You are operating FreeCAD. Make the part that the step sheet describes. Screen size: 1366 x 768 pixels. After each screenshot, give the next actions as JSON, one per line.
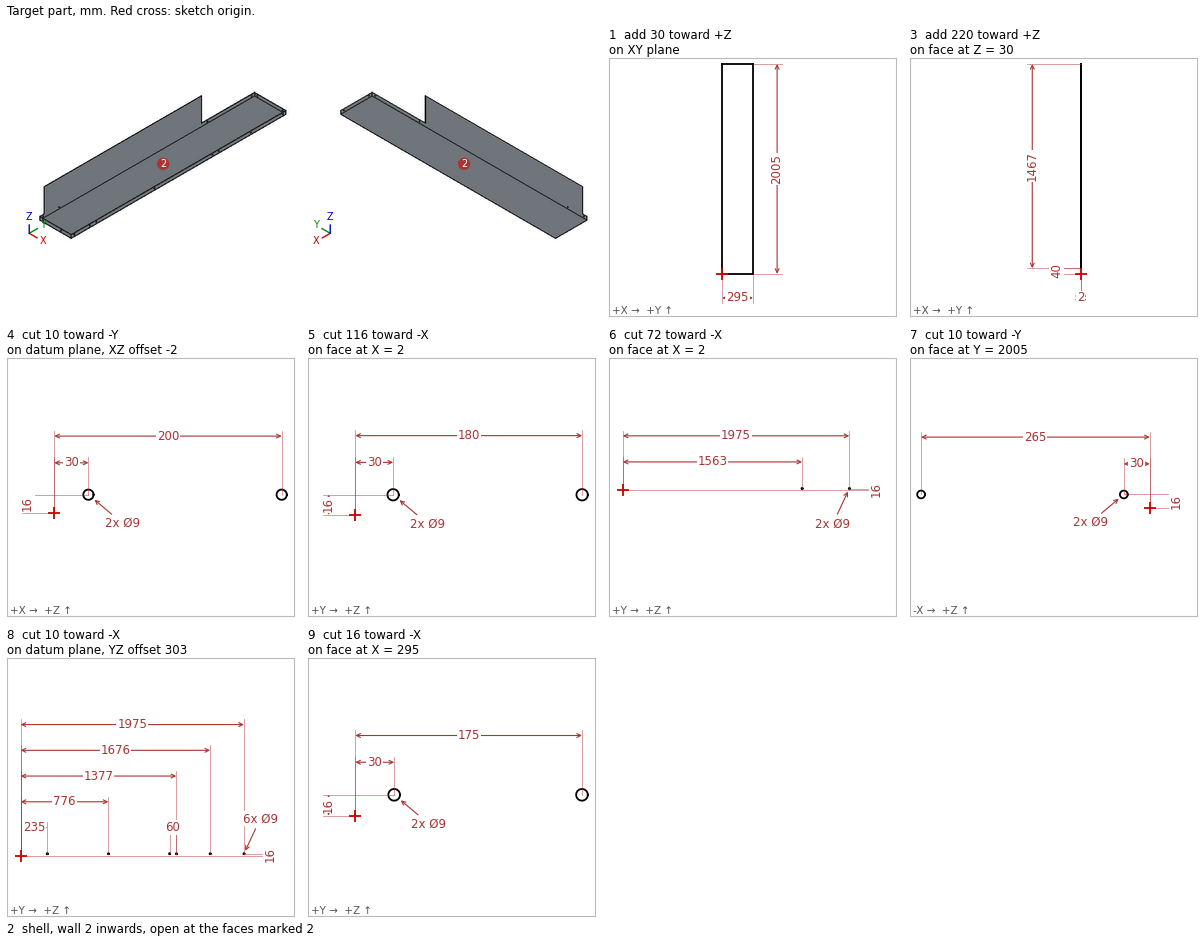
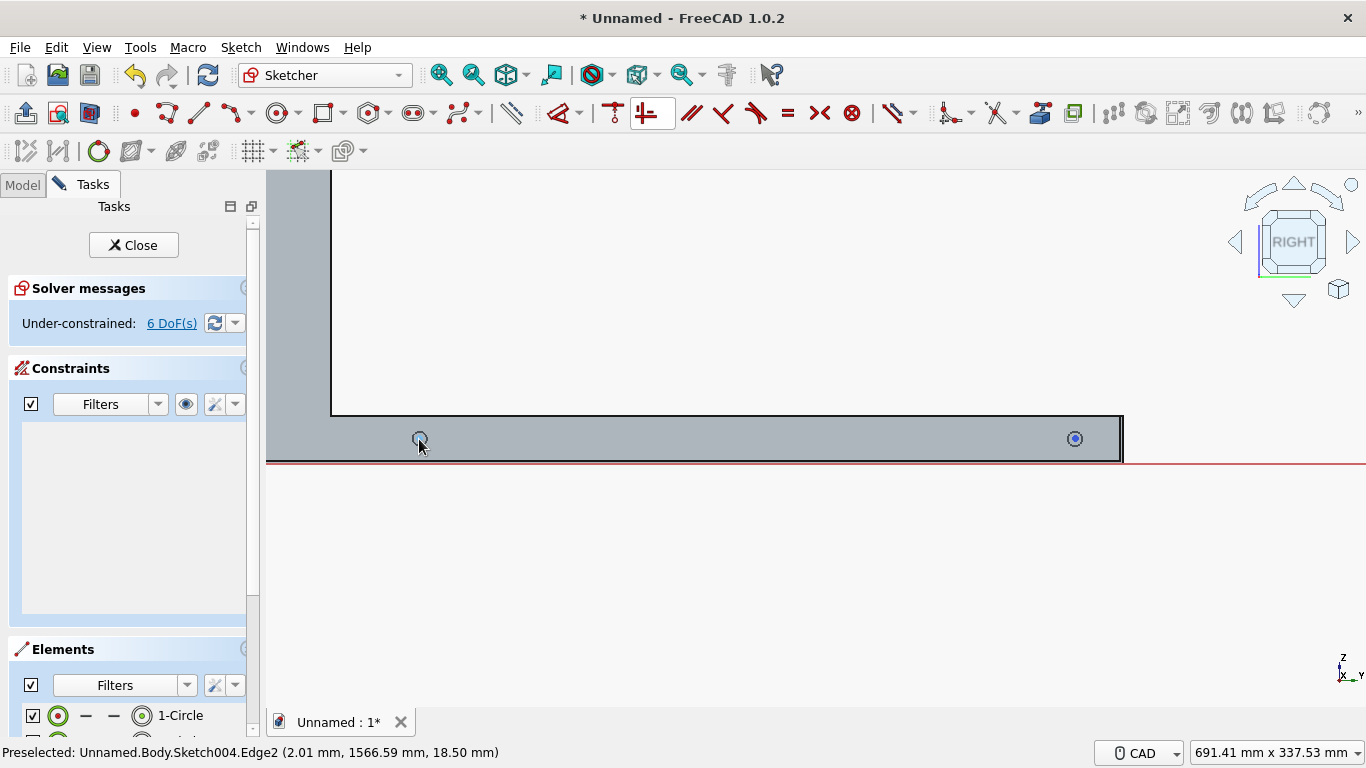
{"action": "scroll", "coordinate": [1080, 434], "scroll_direction": "up", "scroll_amount": 4}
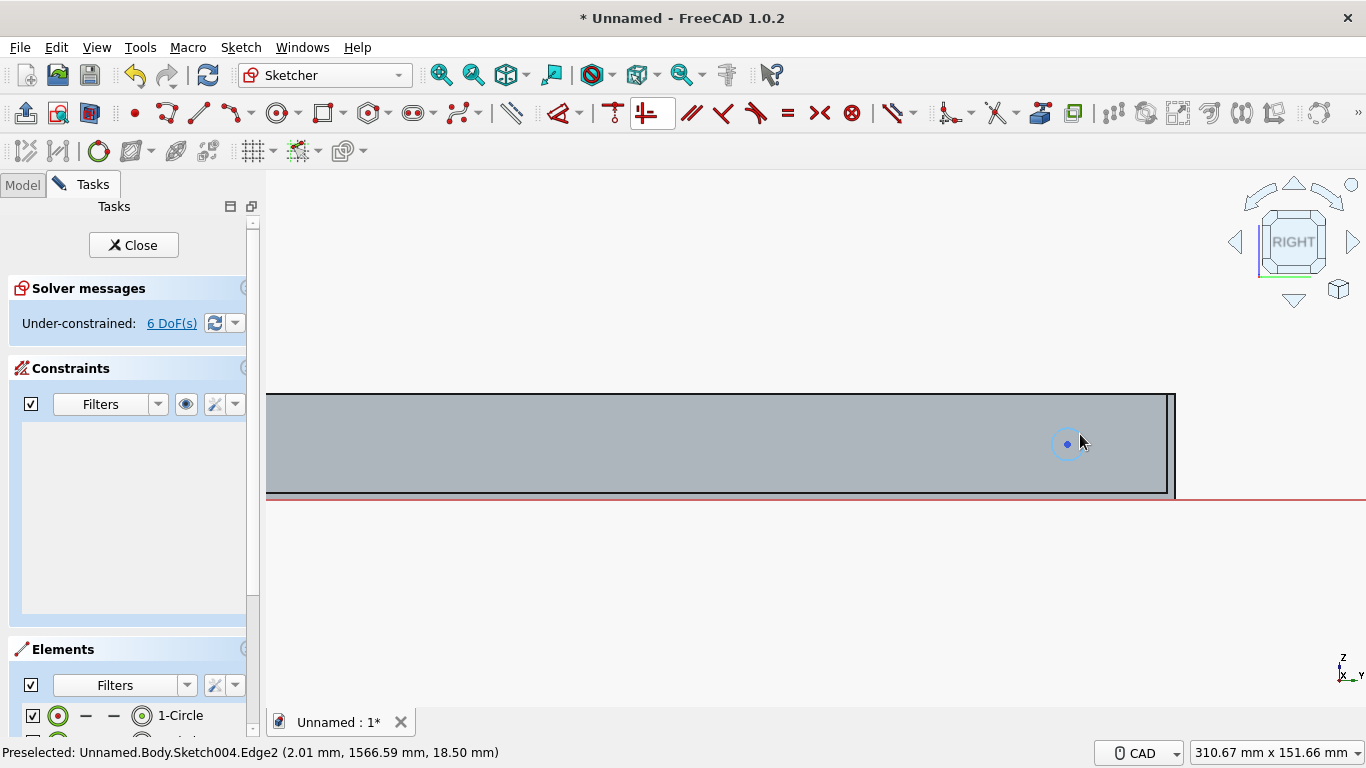
{"action": "left_click", "coordinate": [1079, 433]}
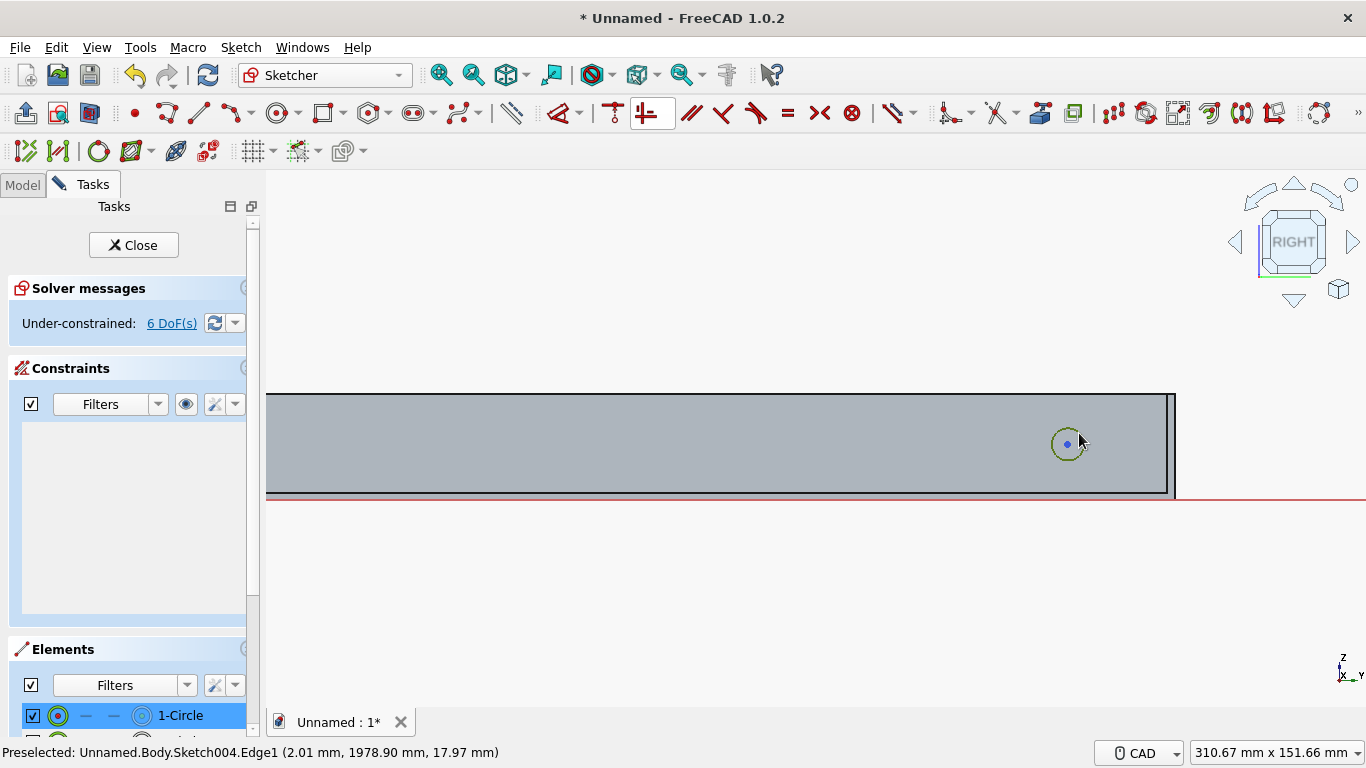
{"action": "scroll", "coordinate": [1081, 434], "scroll_direction": "down", "scroll_amount": 4}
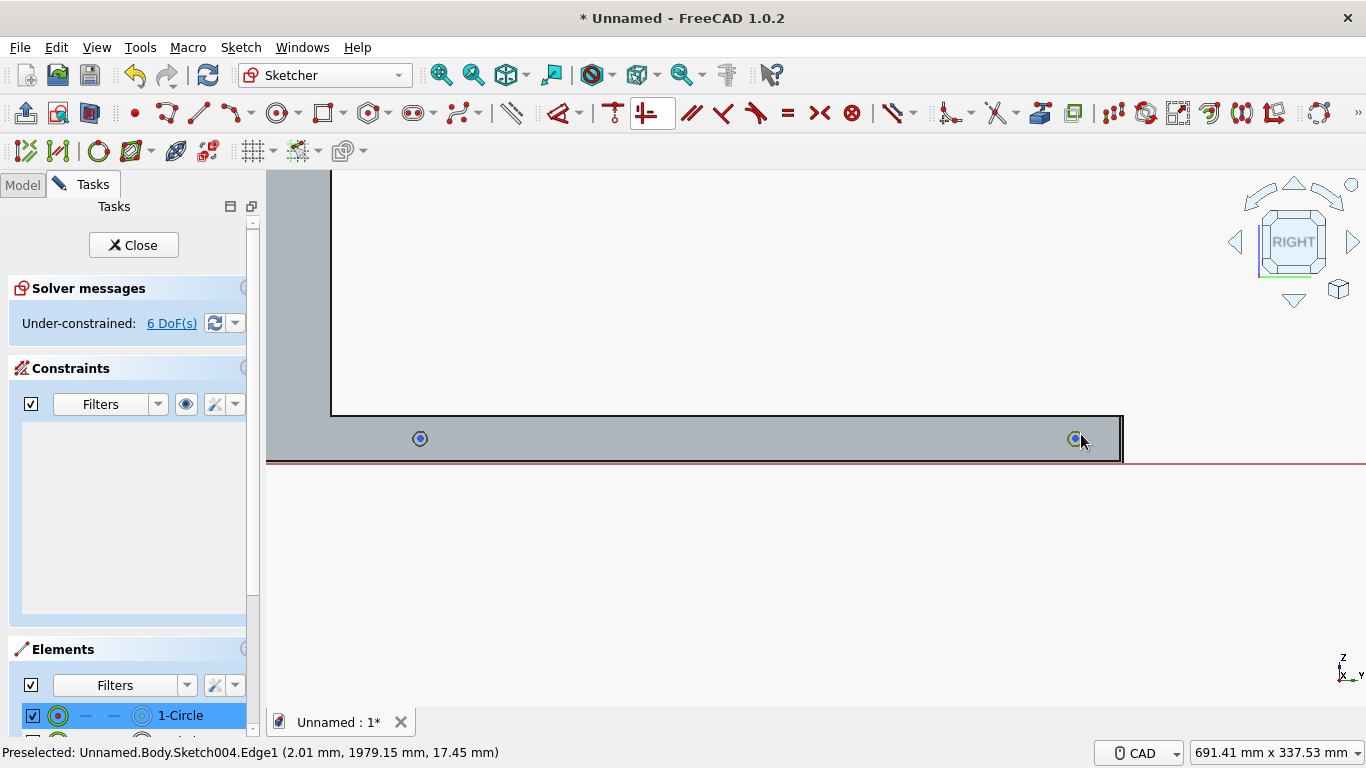
{"action": "scroll", "coordinate": [425, 434], "scroll_direction": "up", "scroll_amount": 4}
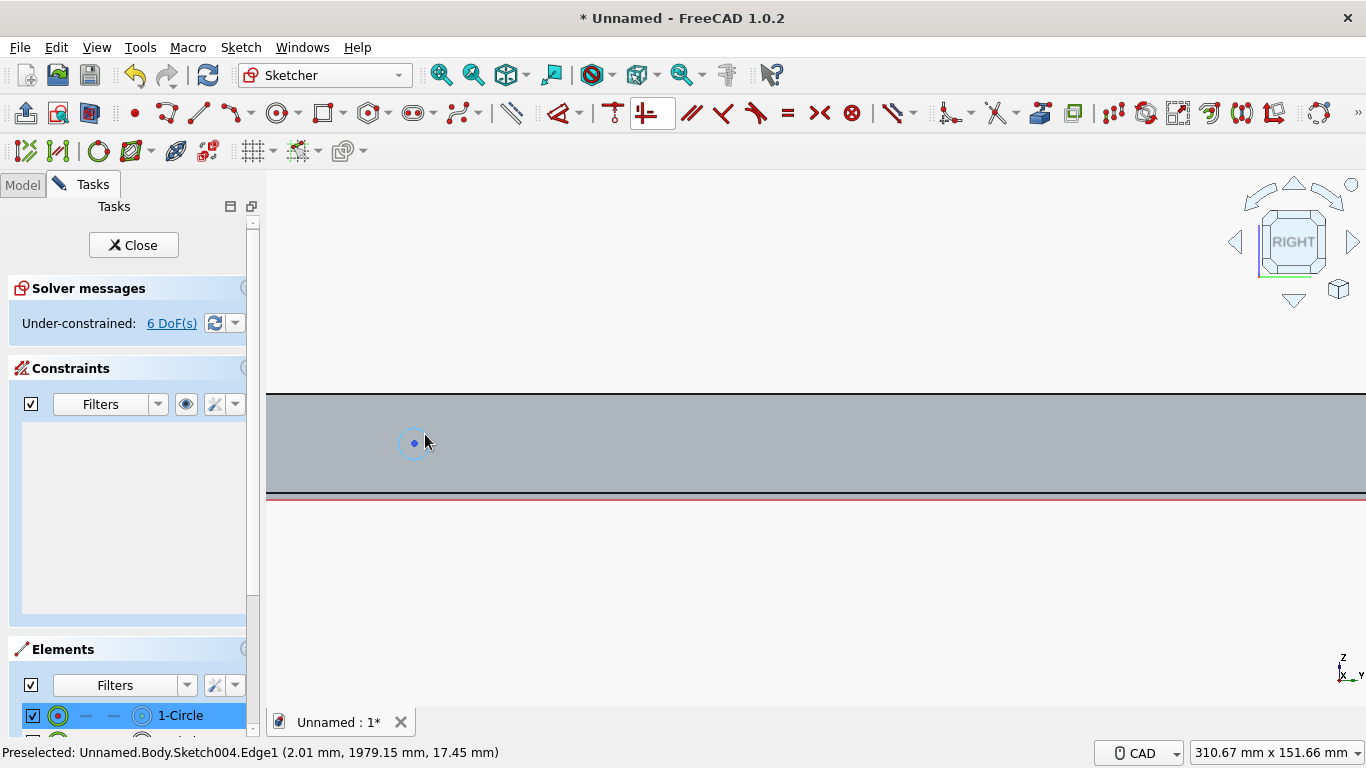
{"action": "left_click", "coordinate": [425, 433]}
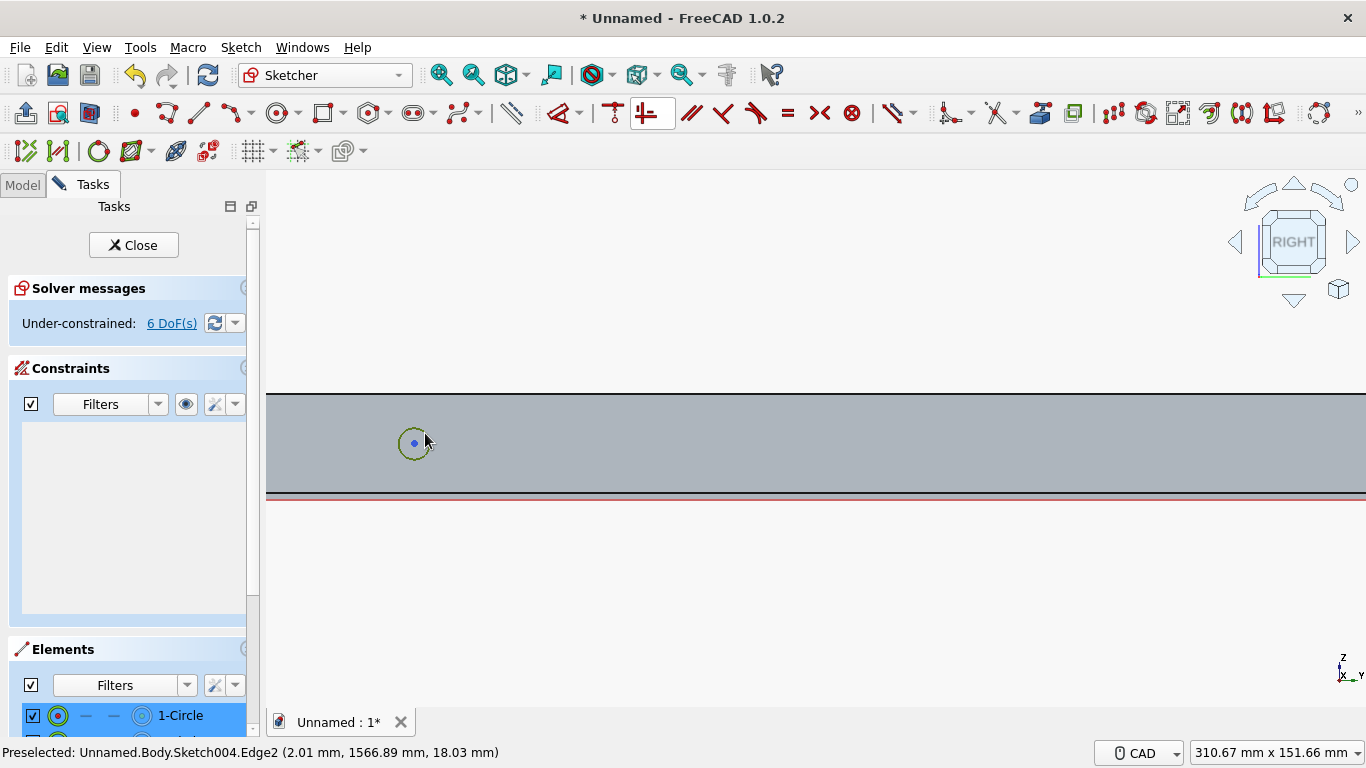
{"action": "left_click", "coordinate": [788, 114]}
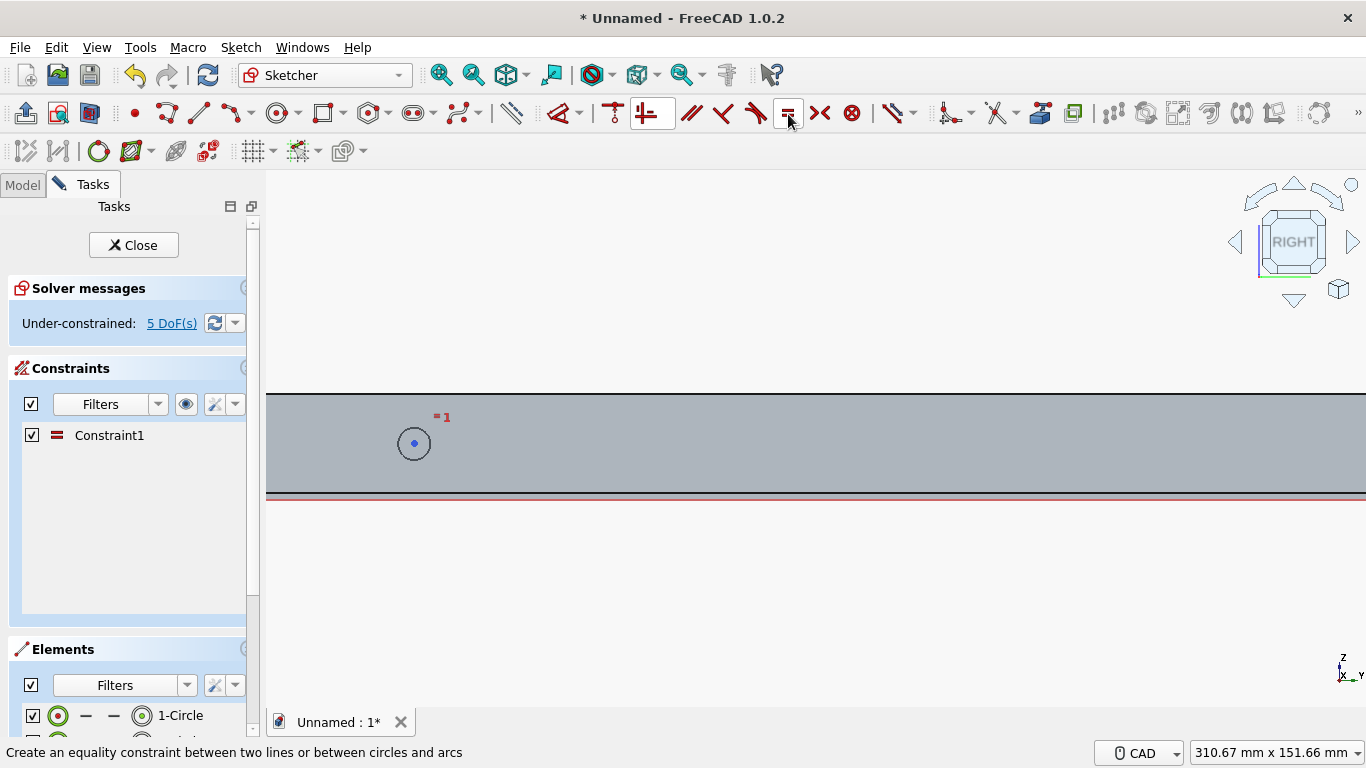
{"action": "scroll", "coordinate": [424, 434], "scroll_direction": "down", "scroll_amount": 4}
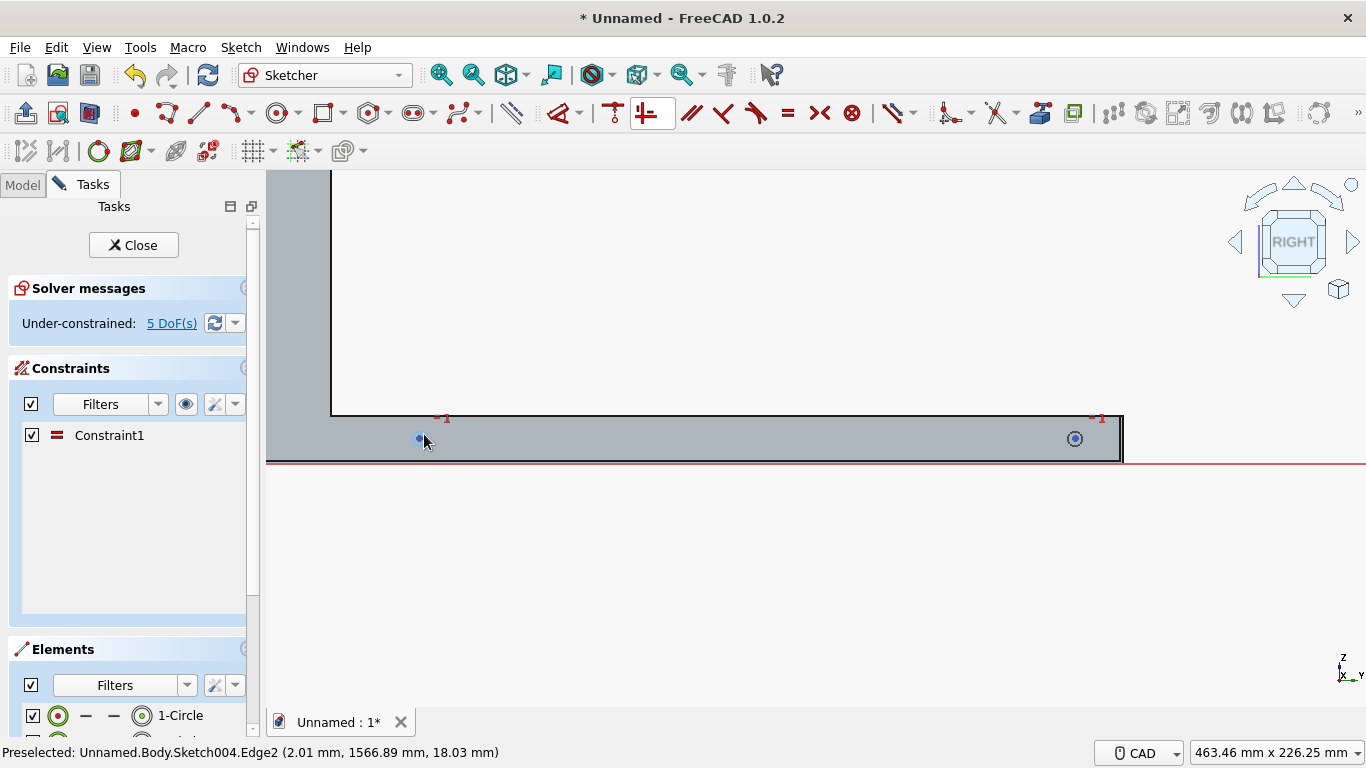
{"action": "left_click", "coordinate": [1075, 439]}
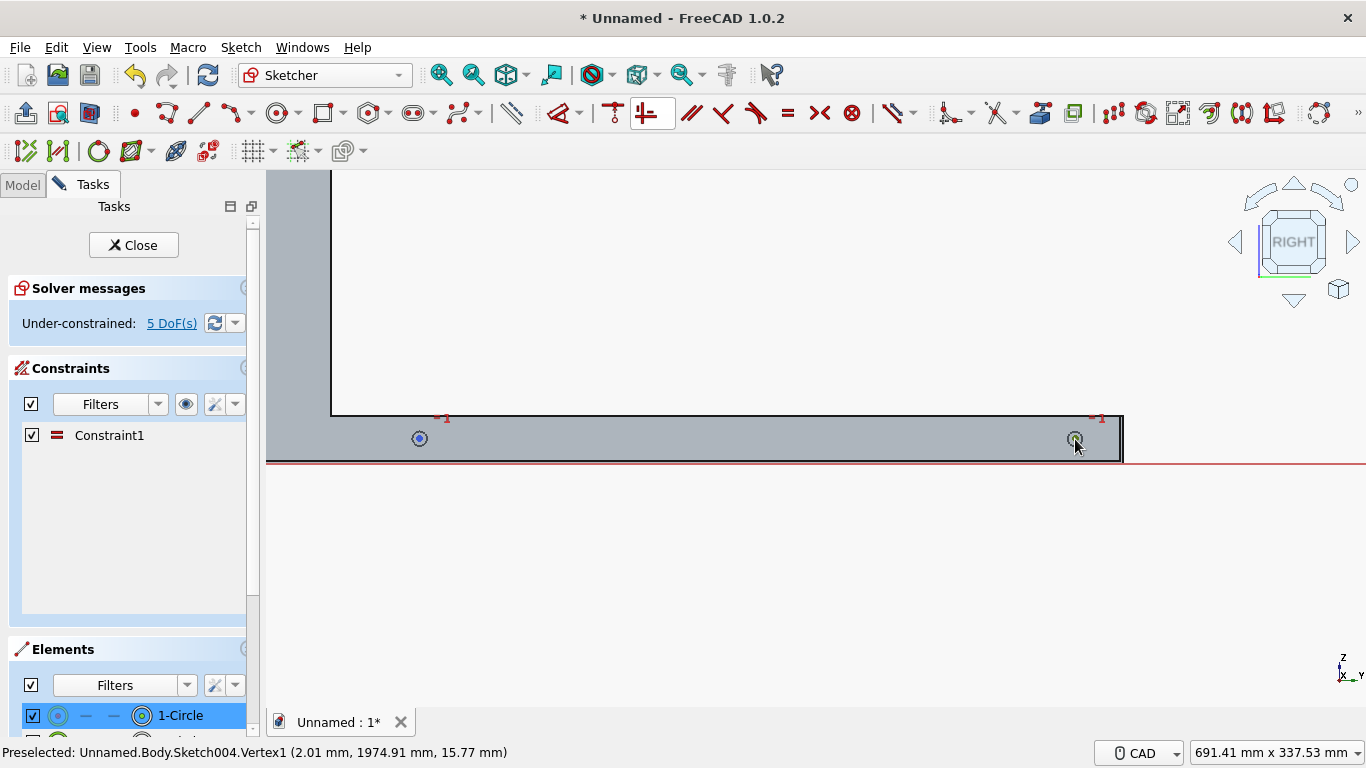
{"action": "left_click", "coordinate": [420, 439]}